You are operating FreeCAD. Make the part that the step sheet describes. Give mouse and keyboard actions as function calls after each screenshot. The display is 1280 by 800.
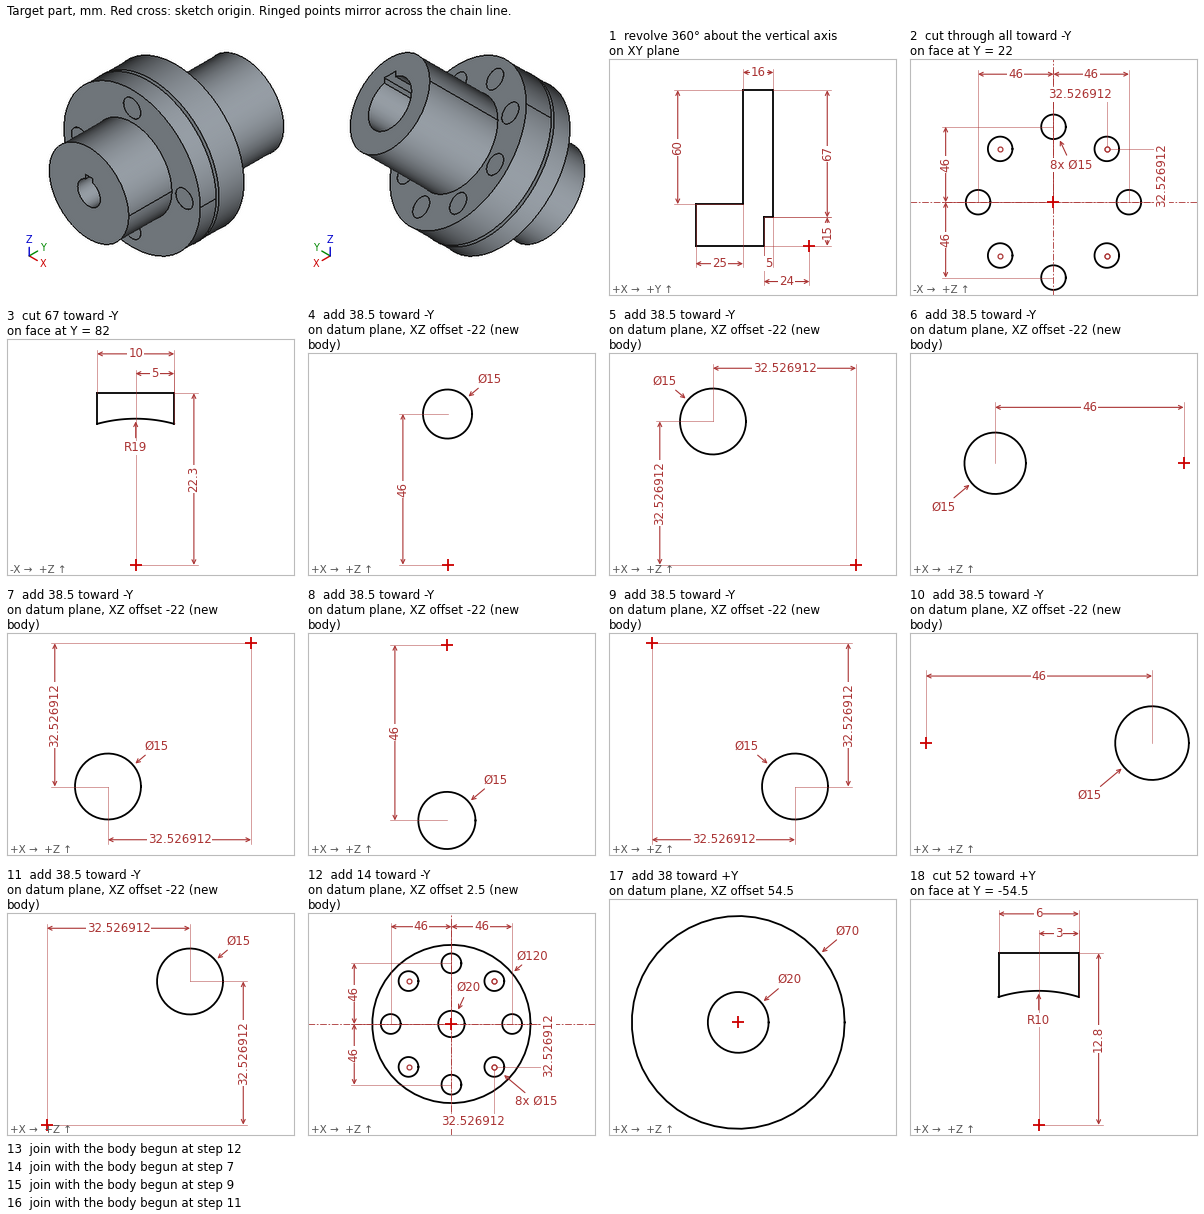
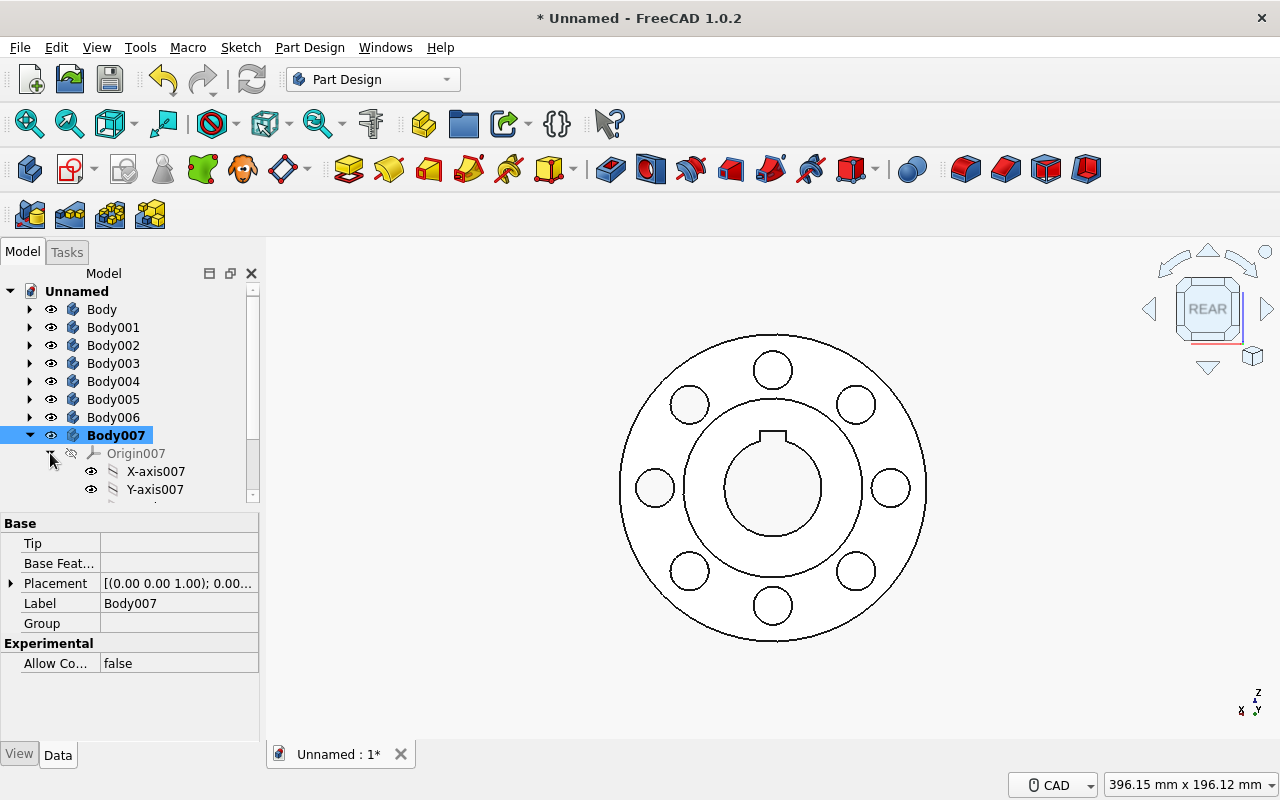
scroll(100, 395, down, 3)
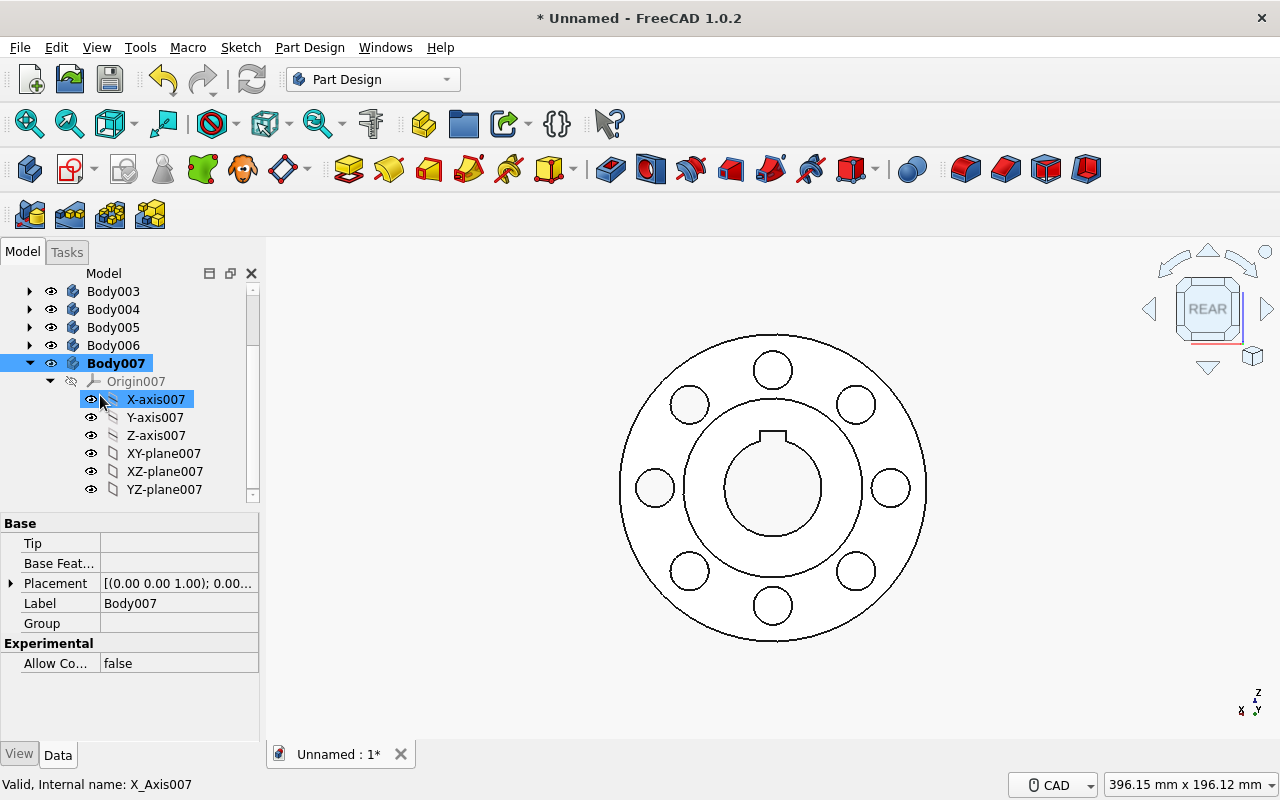
click(136, 471)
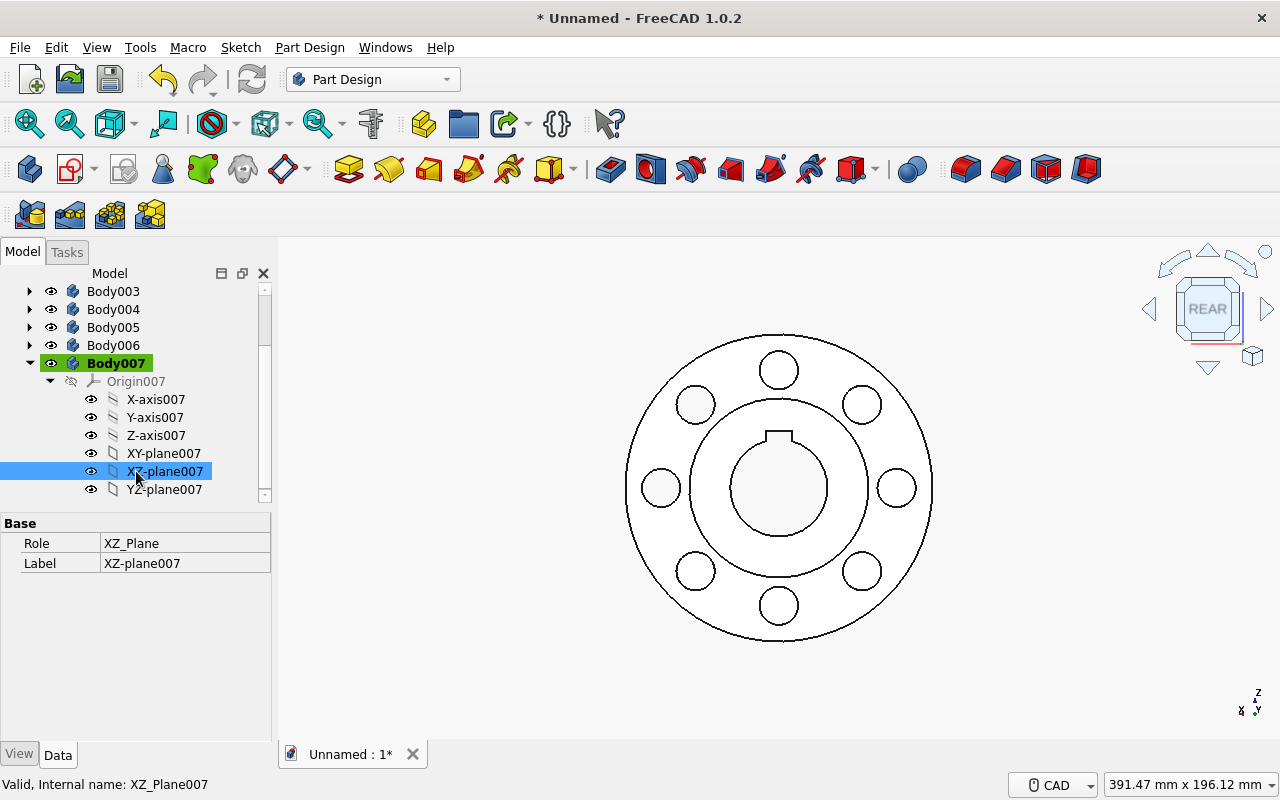
click(284, 170)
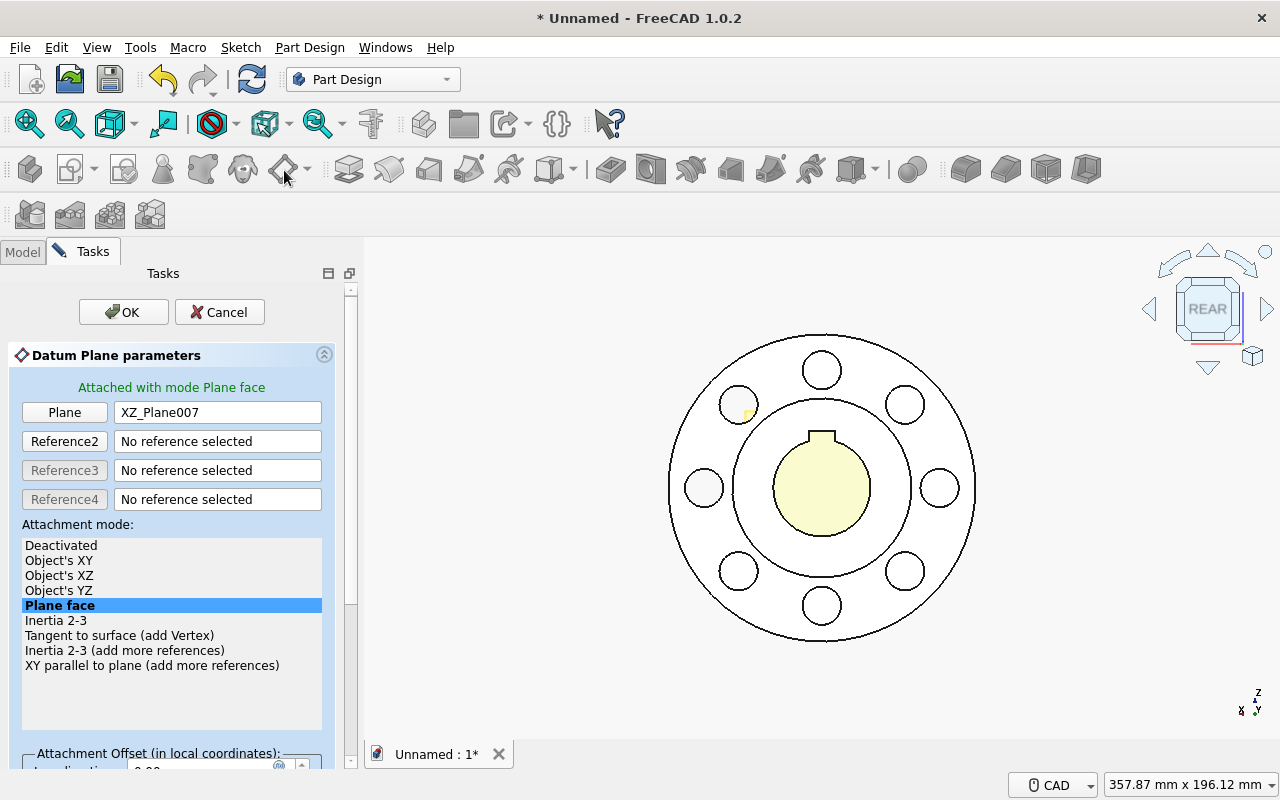
scroll(351, 526, down, 3)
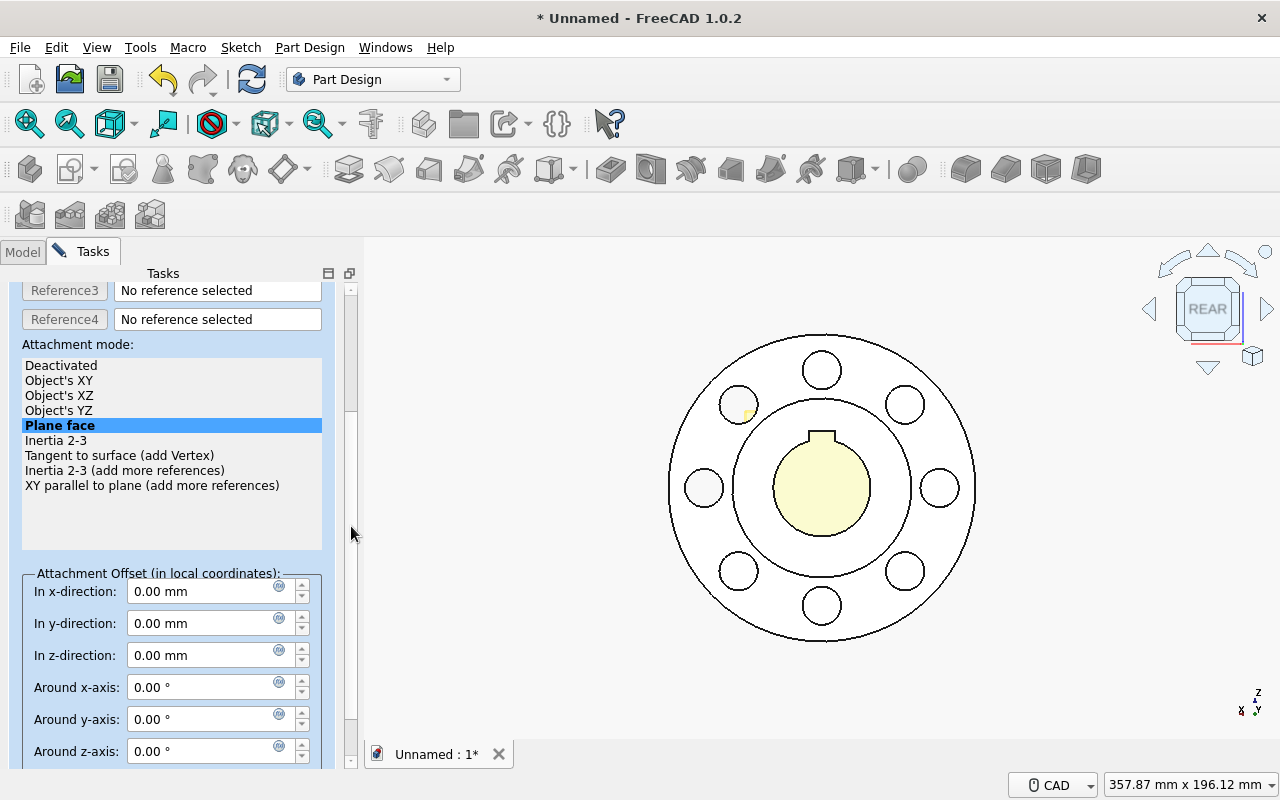
triple_click(210, 655)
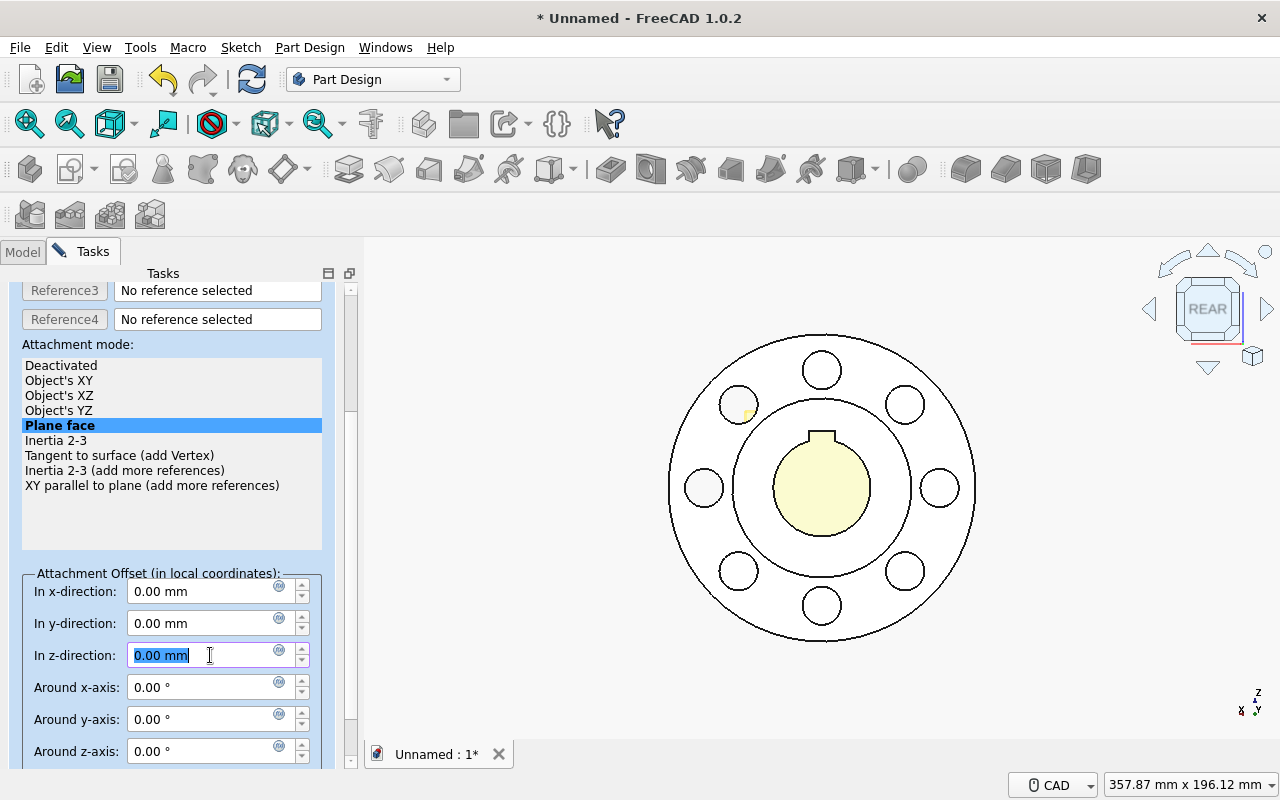
text(-22)
key(Tab)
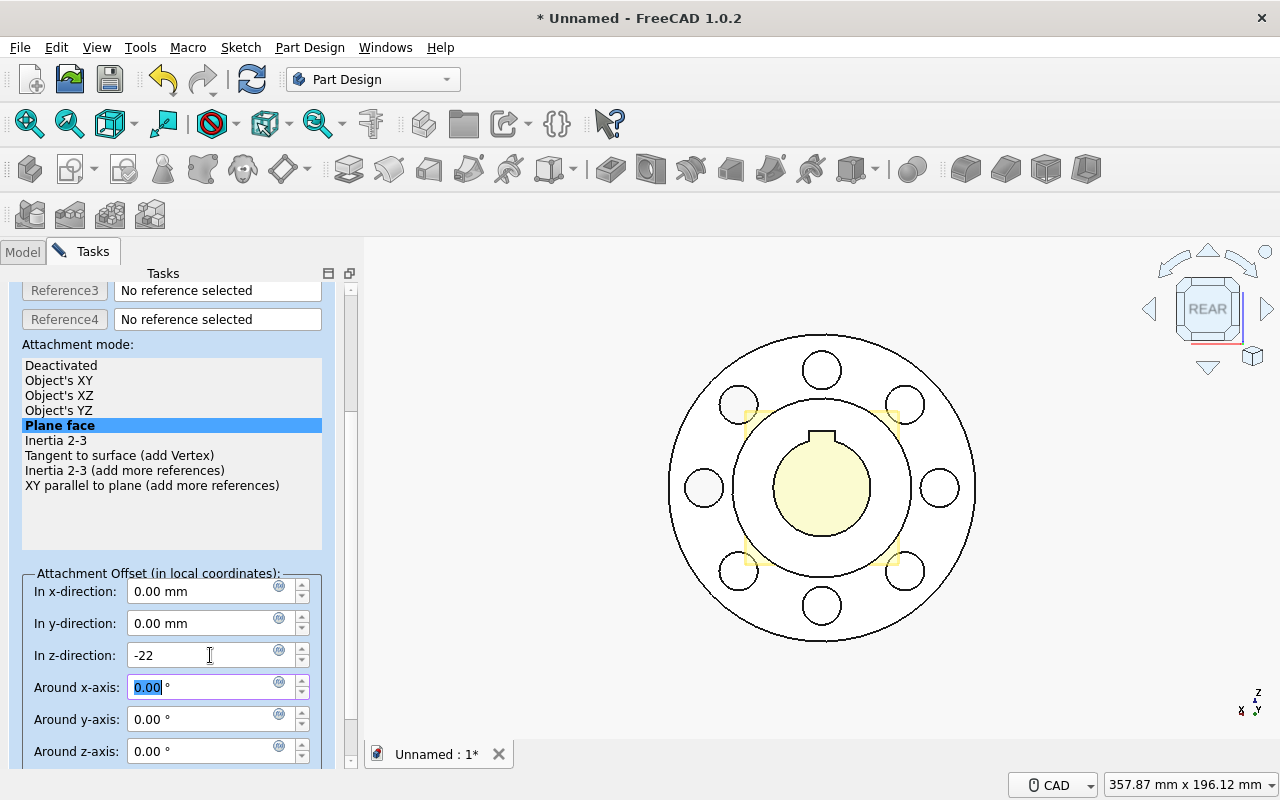
scroll(351, 526, up, 4)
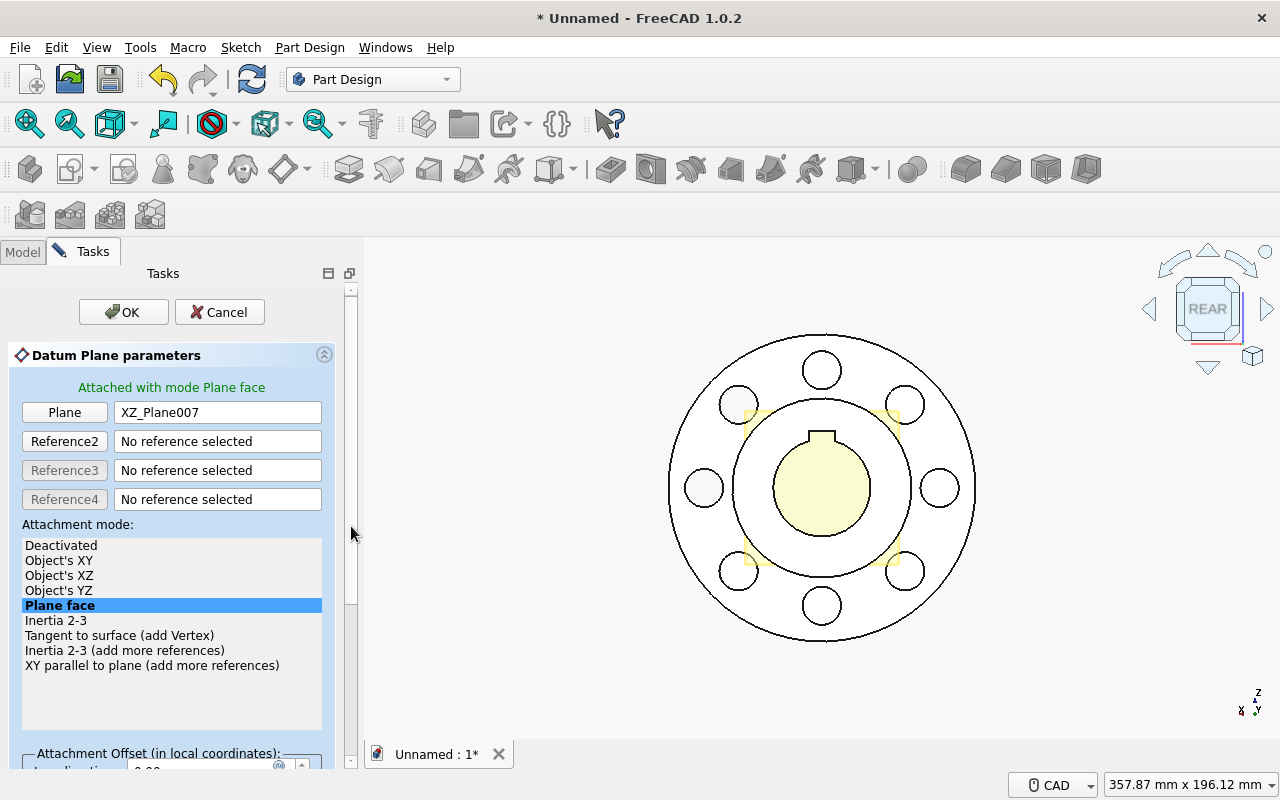
click(124, 312)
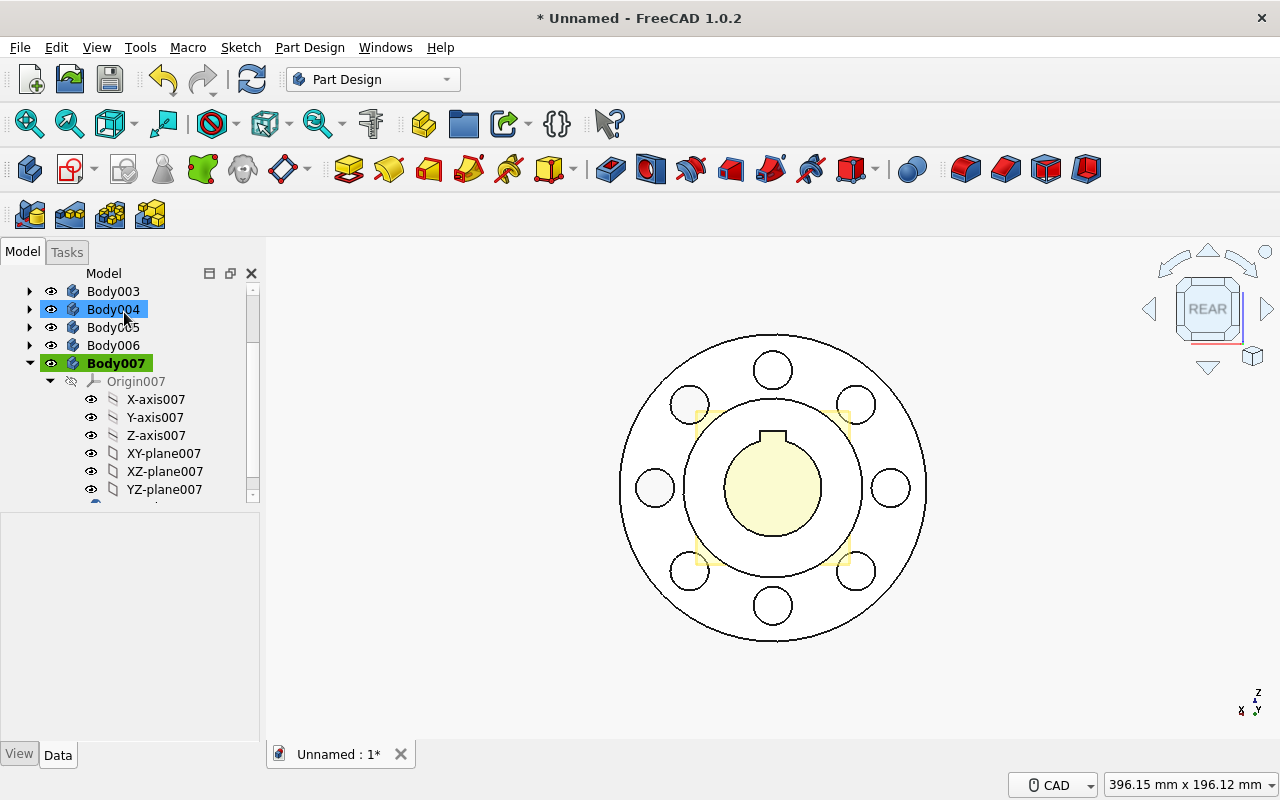
scroll(120, 395, down, 3)